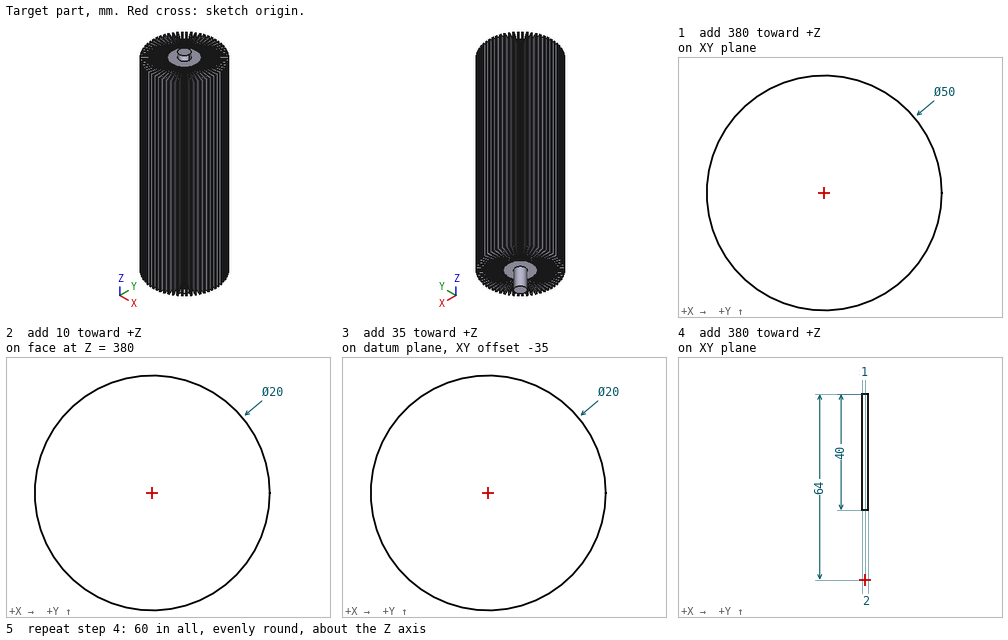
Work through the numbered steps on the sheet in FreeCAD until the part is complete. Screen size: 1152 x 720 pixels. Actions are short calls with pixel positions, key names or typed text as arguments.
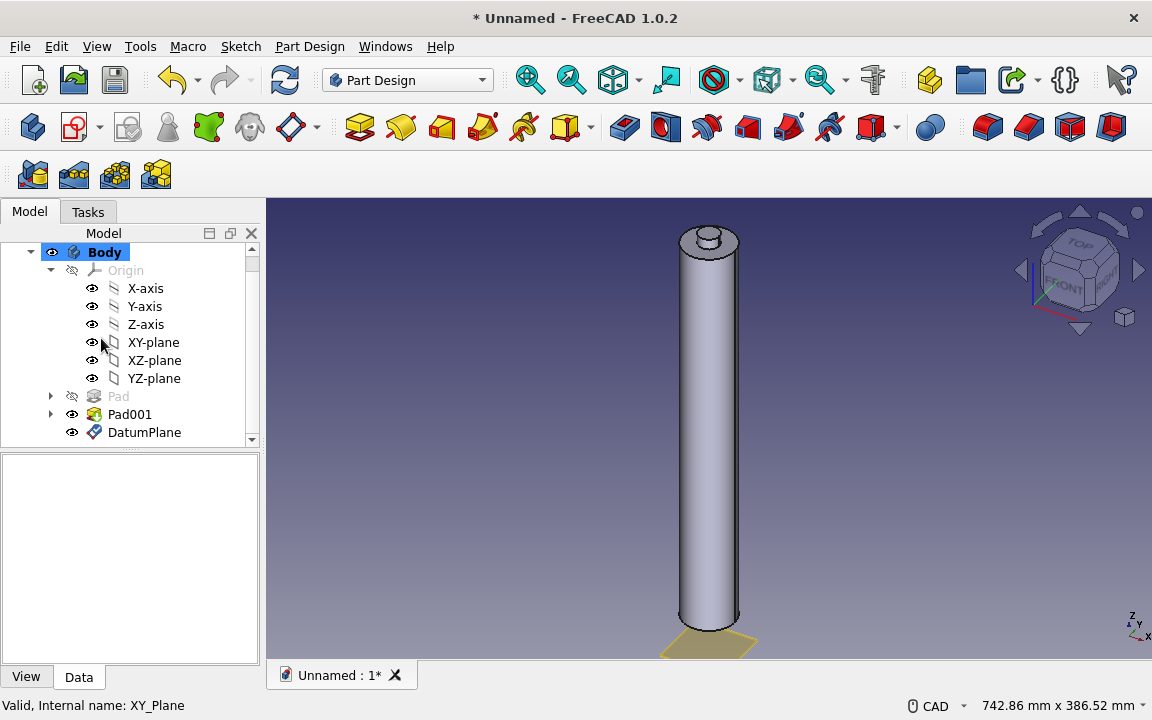
click(117, 432)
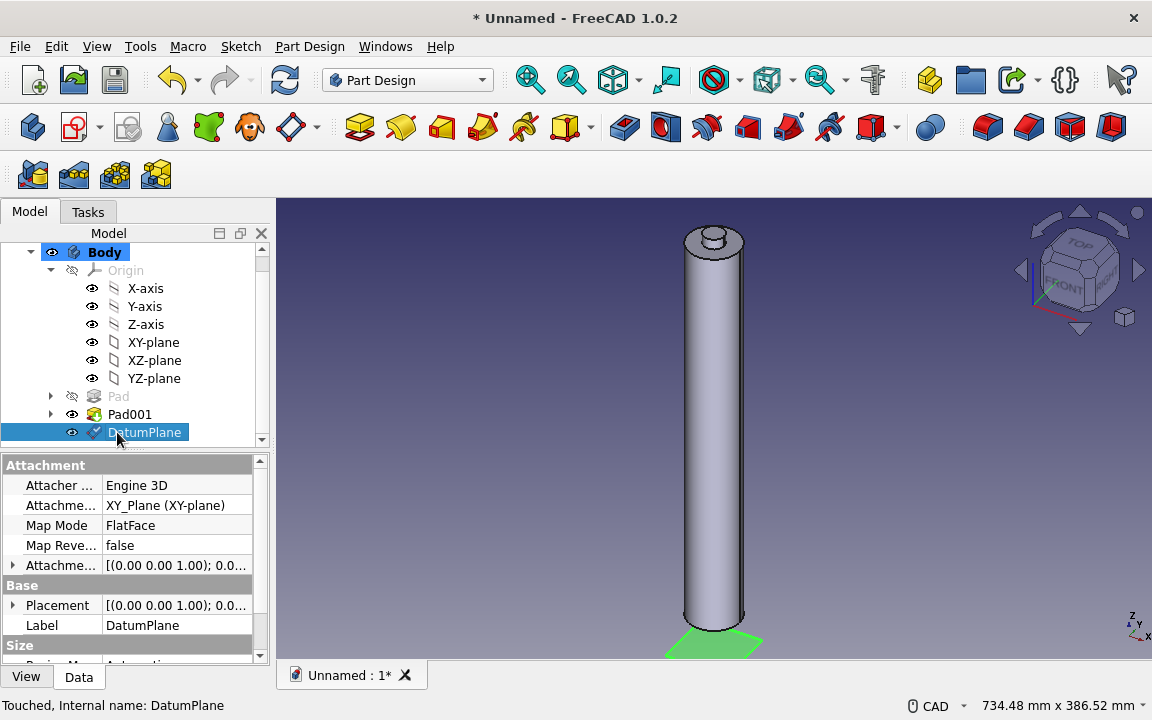
click(74, 128)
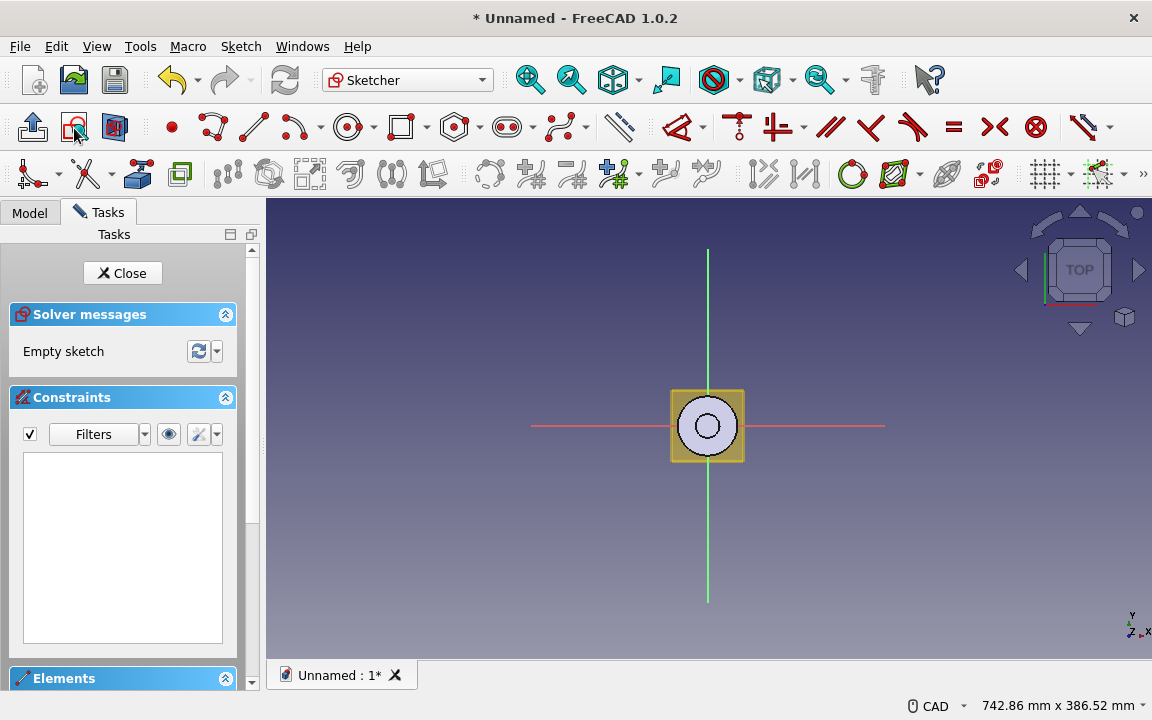
key(q)
key(s)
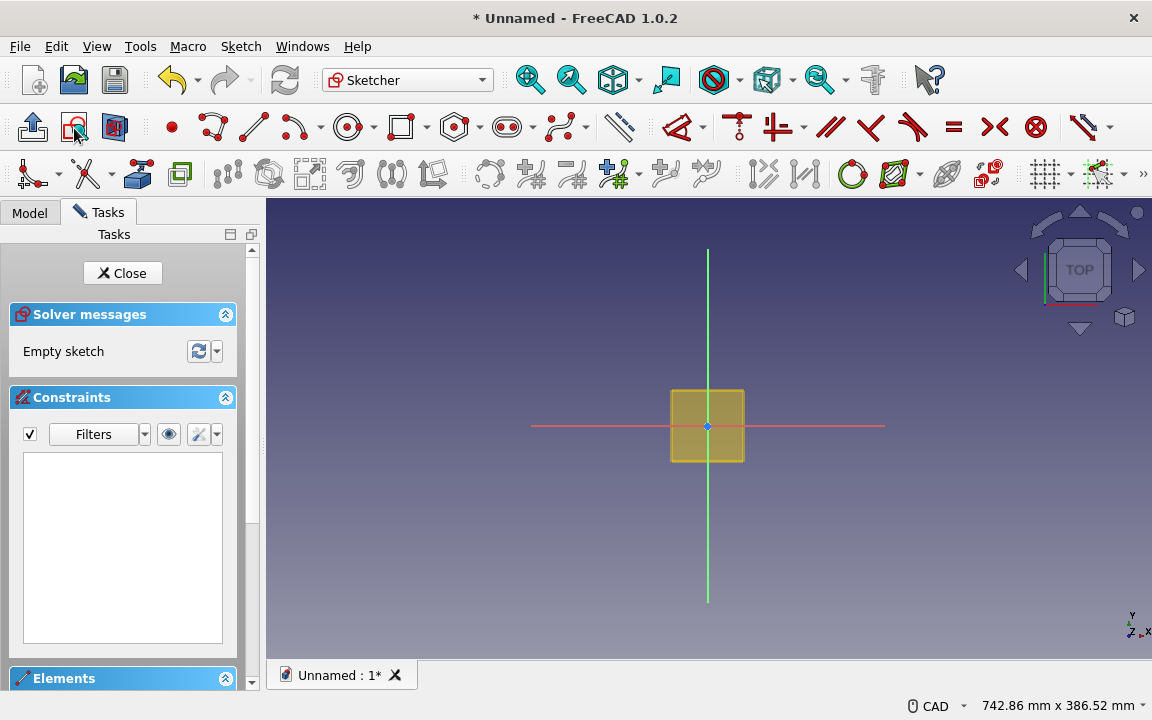
scroll(714, 426, up, 12)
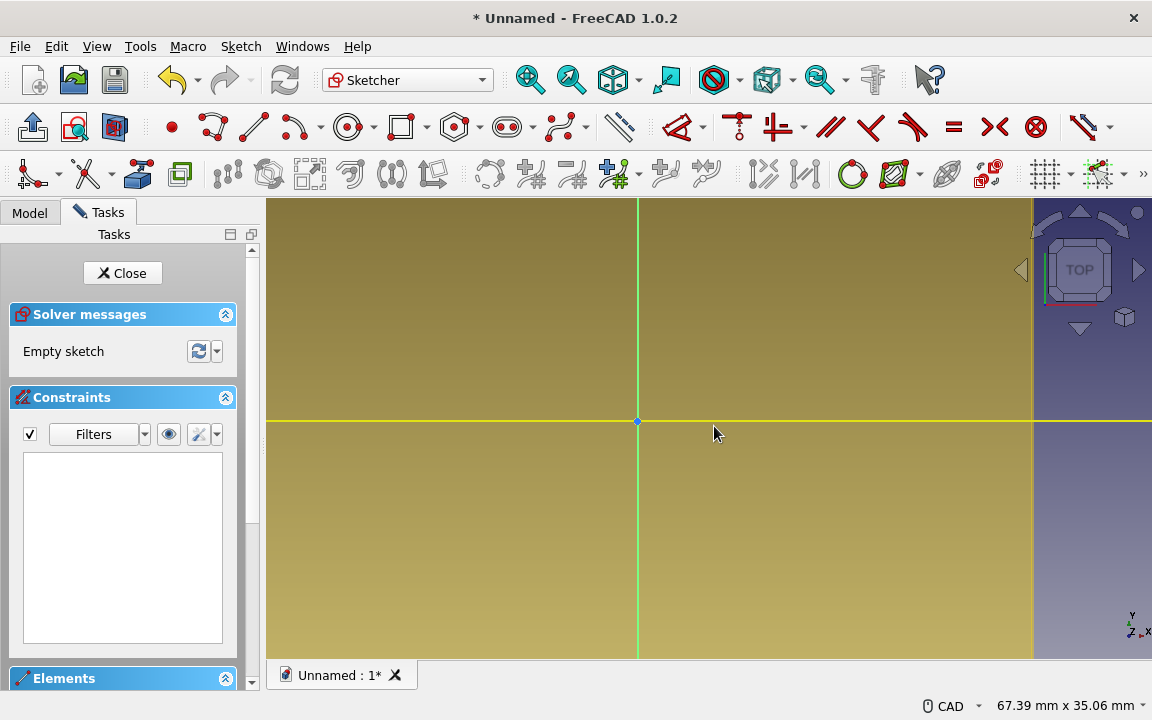
key(g)
key(c)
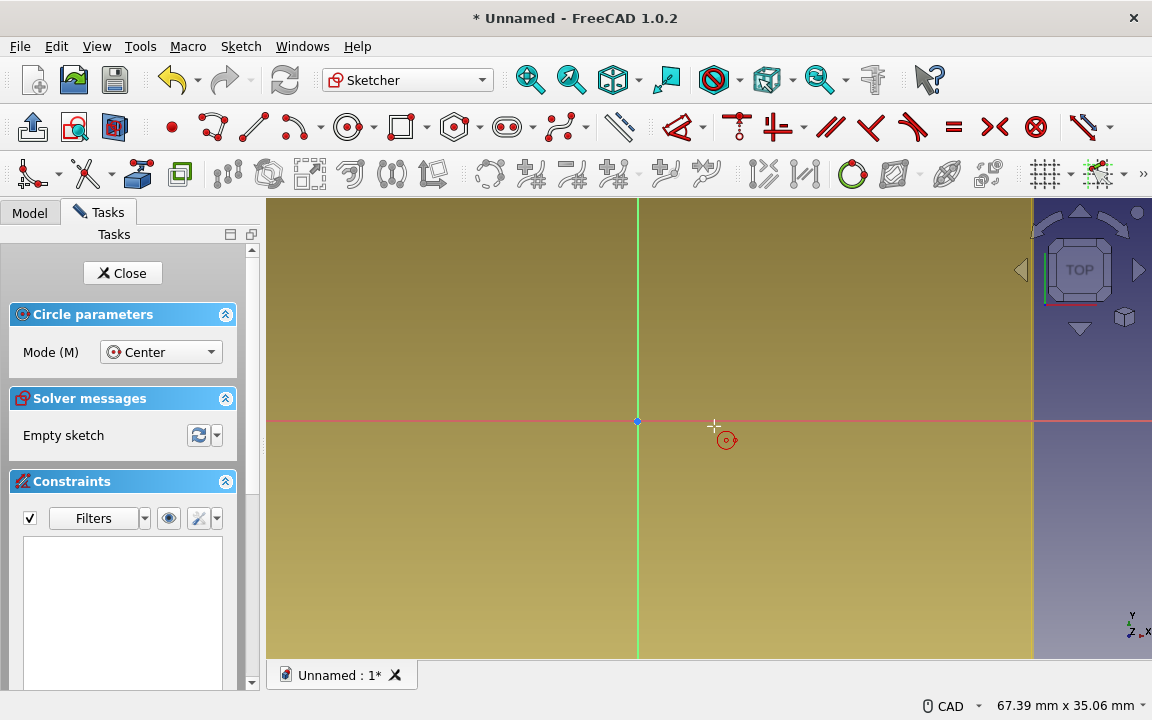
click(638, 421)
click(731, 328)
key(Escape)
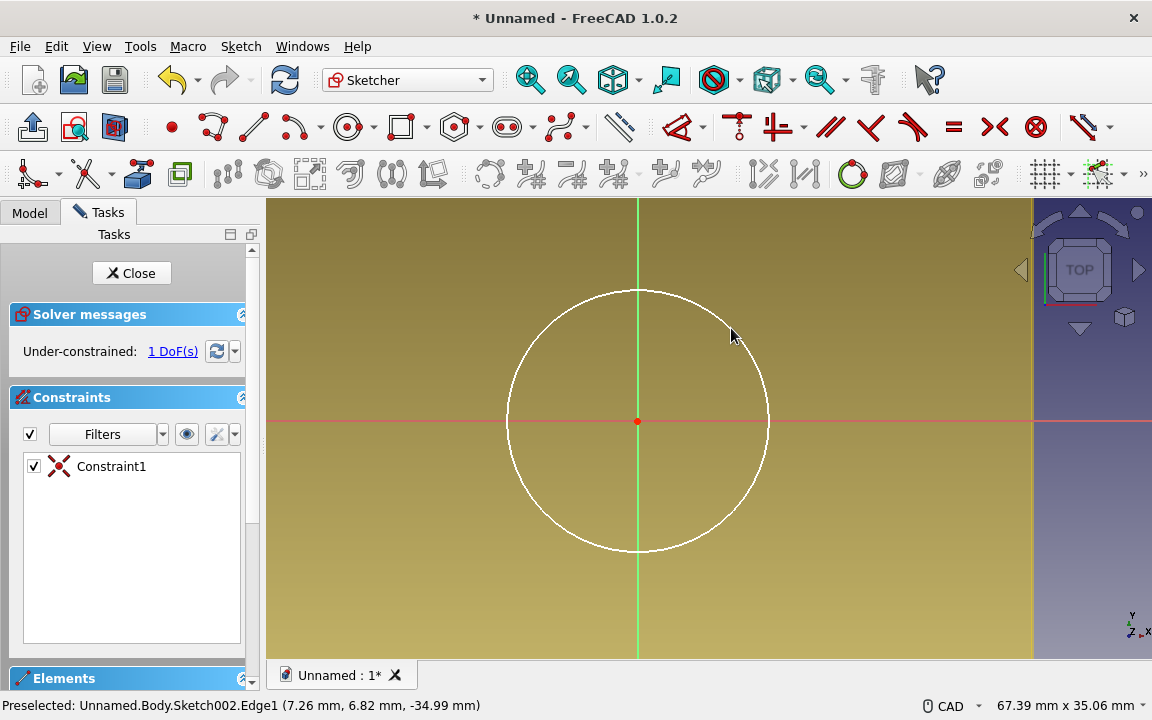
click(676, 128)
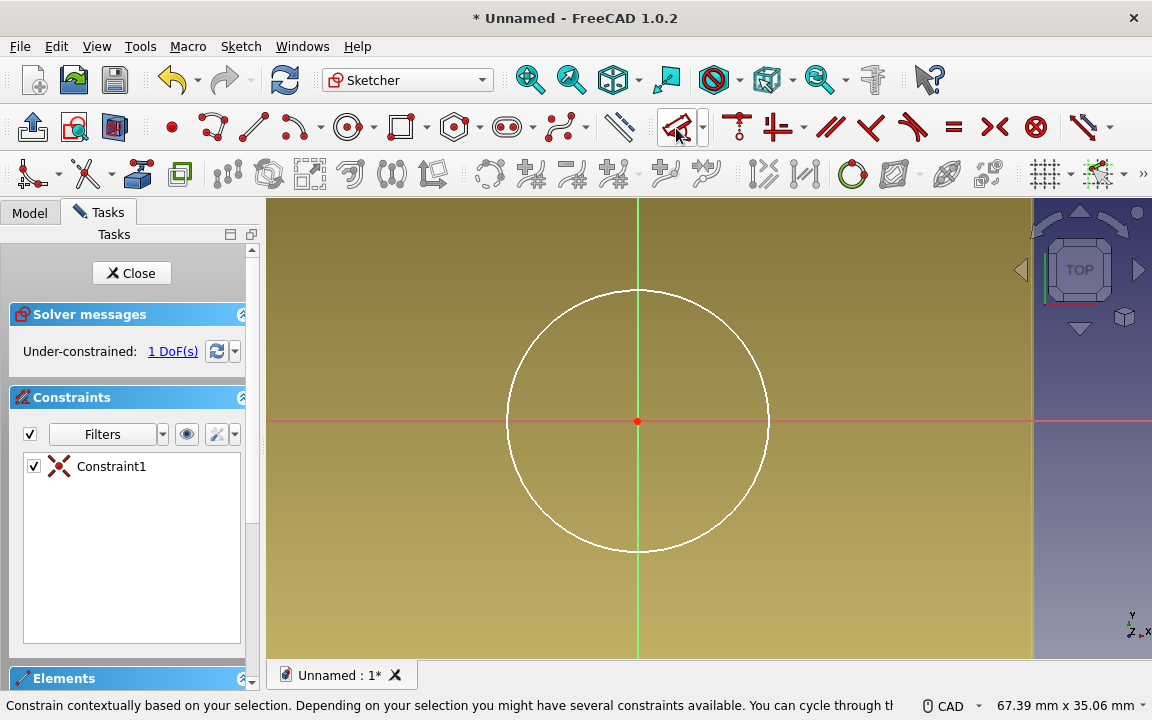
click(730, 328)
click(752, 305)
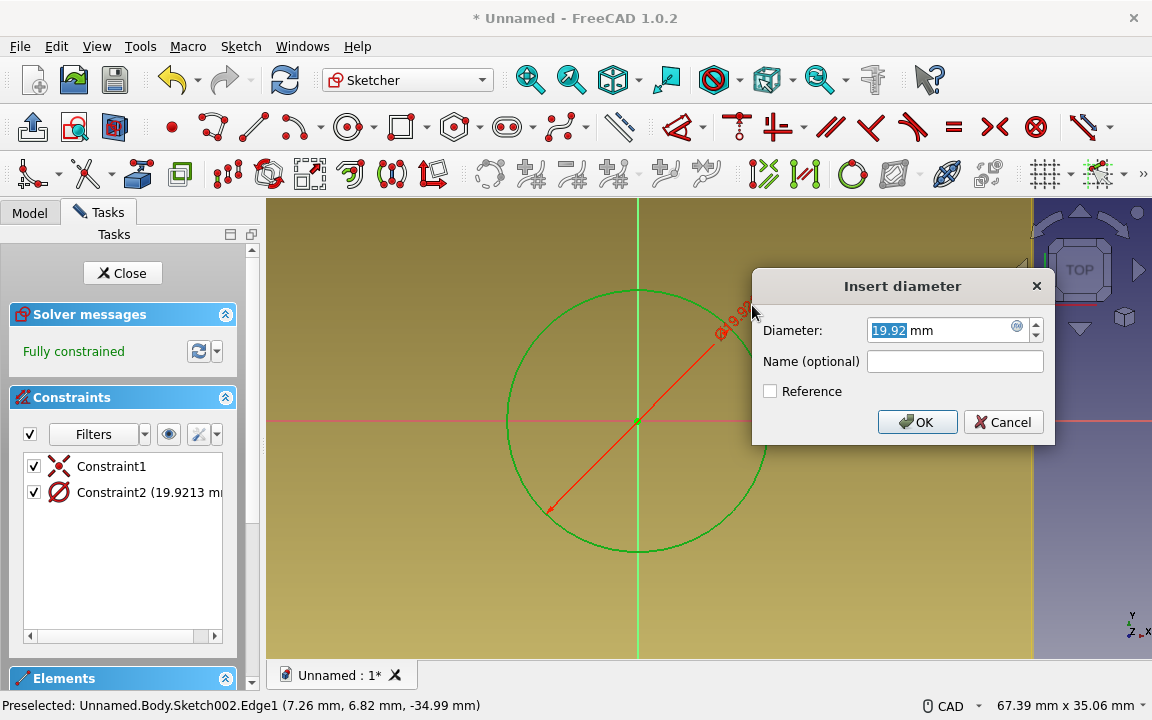
text(20)
key(Return)
key(Escape)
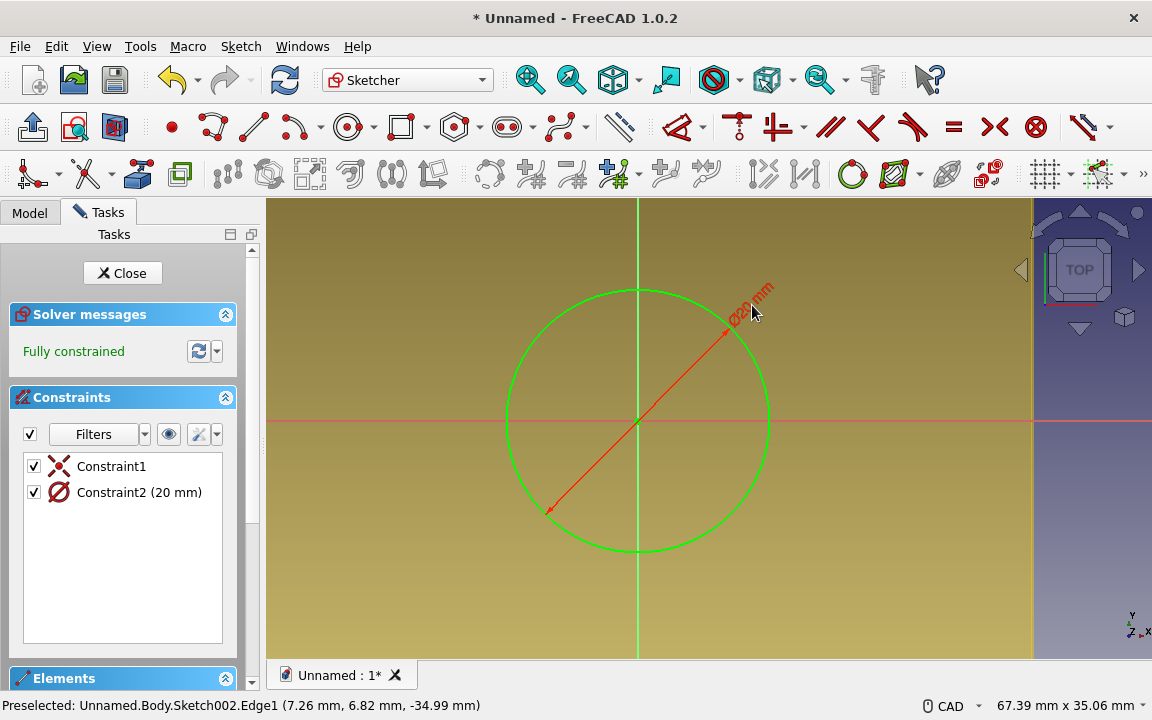
click(123, 273)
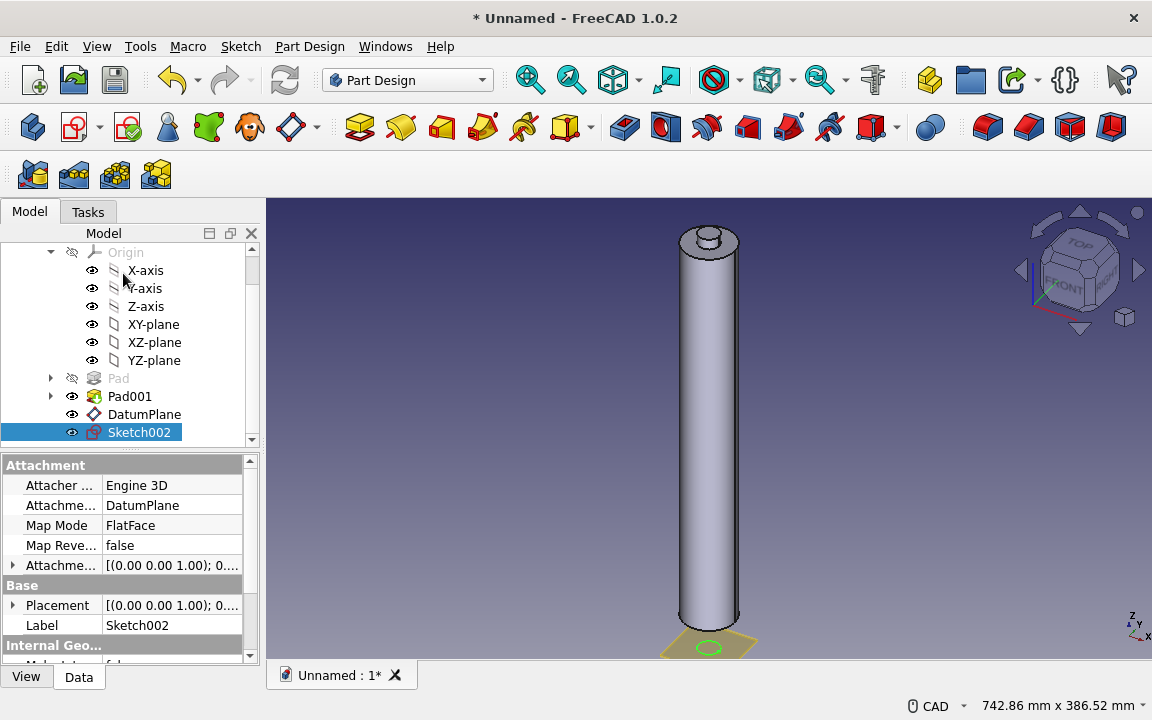
click(360, 128)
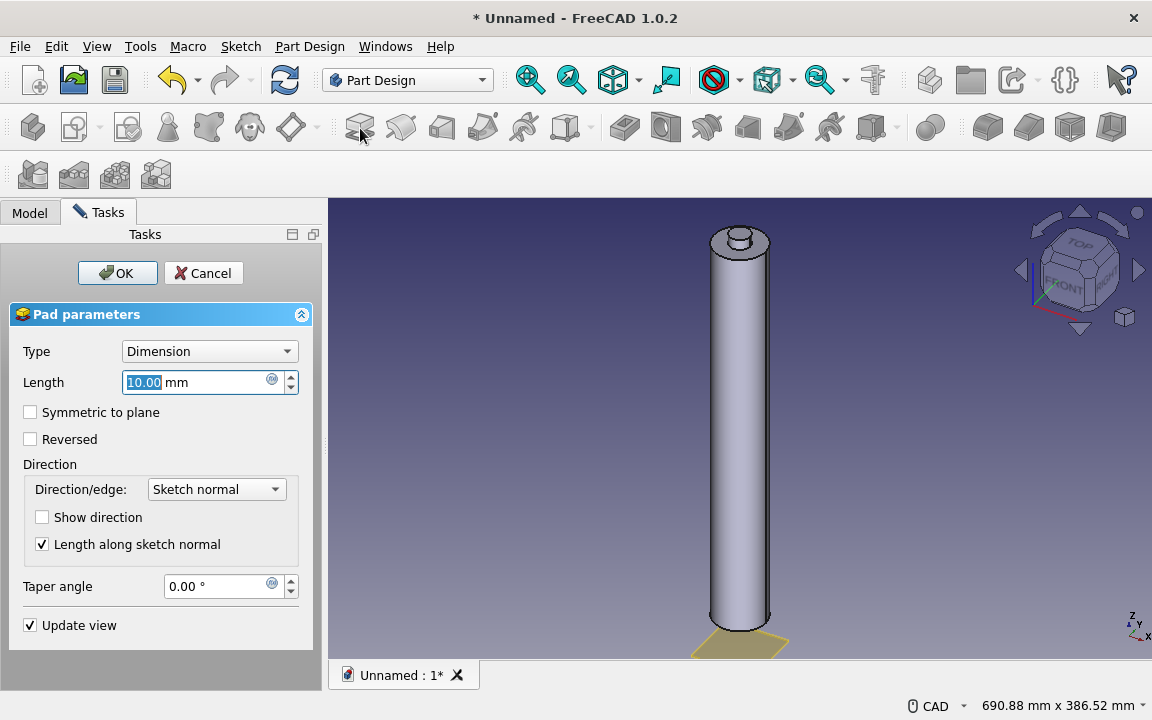
text(35)
key(Tab)